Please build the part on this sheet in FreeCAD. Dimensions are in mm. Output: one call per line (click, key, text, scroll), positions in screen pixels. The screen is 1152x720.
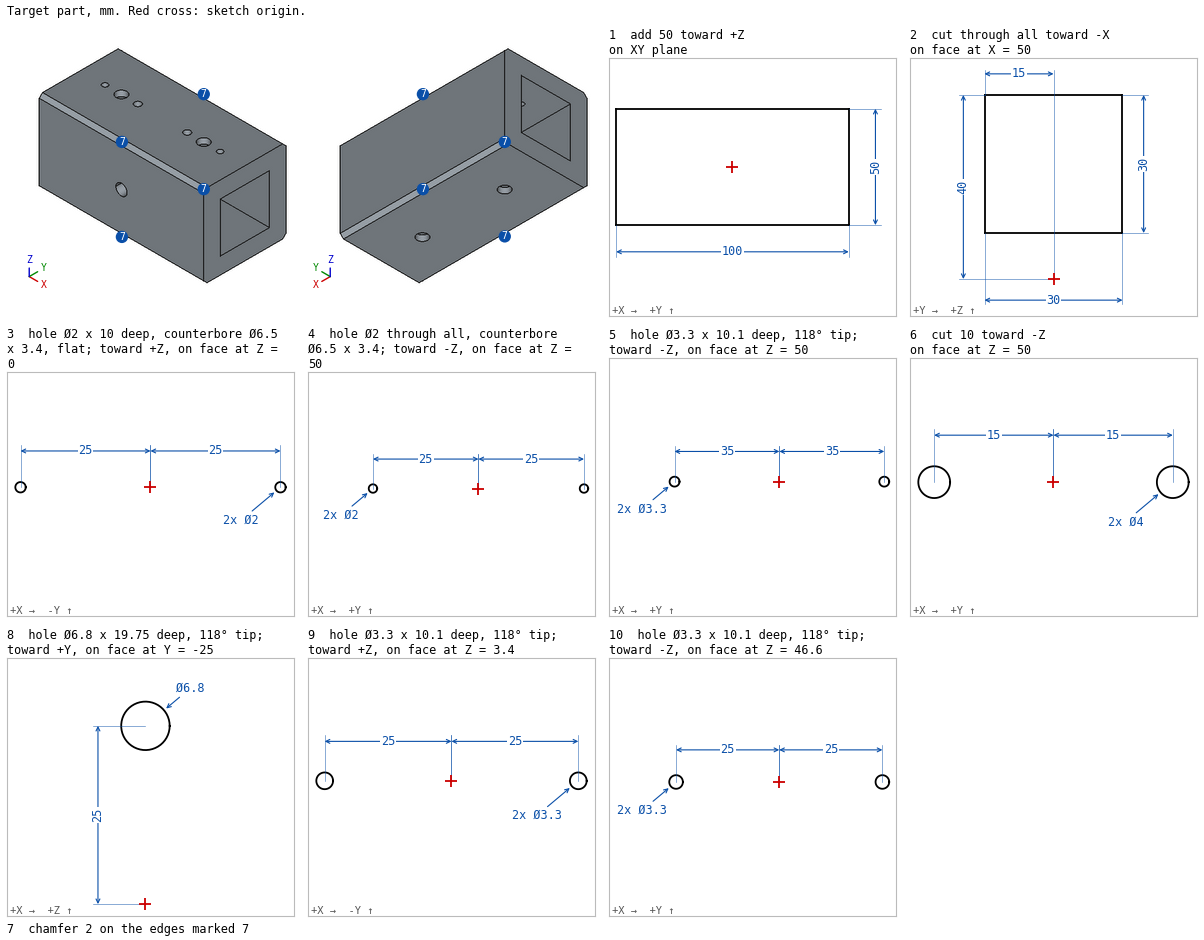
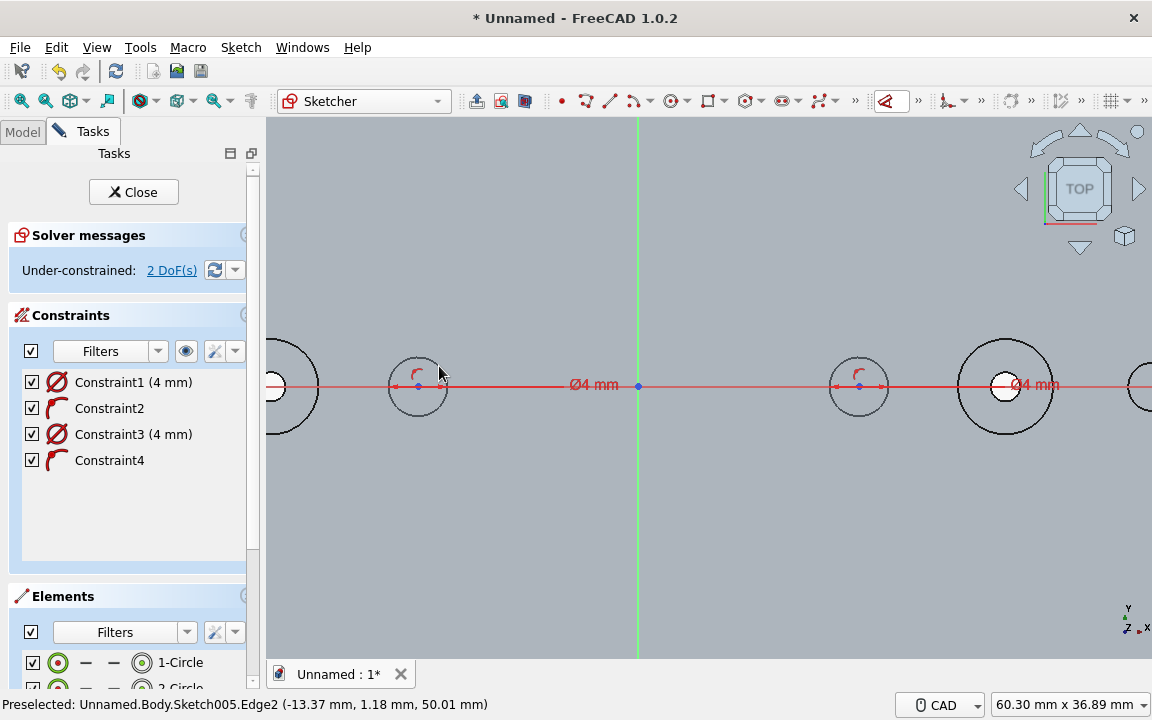
click(859, 387)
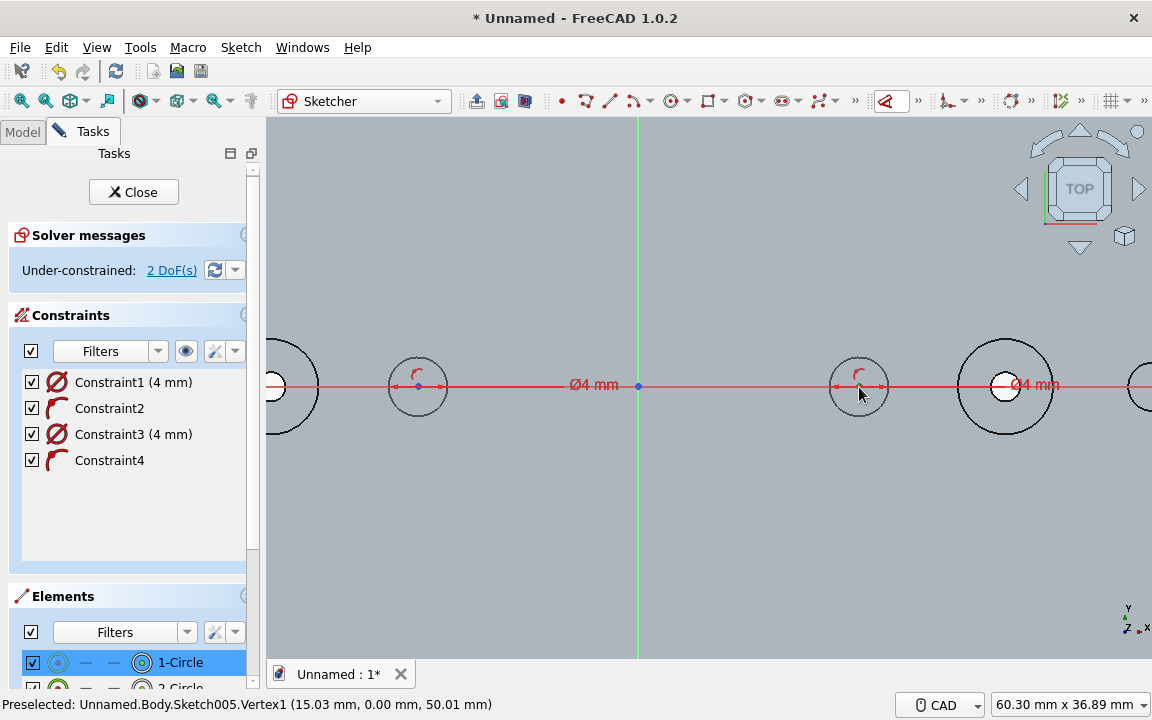
click(904, 102)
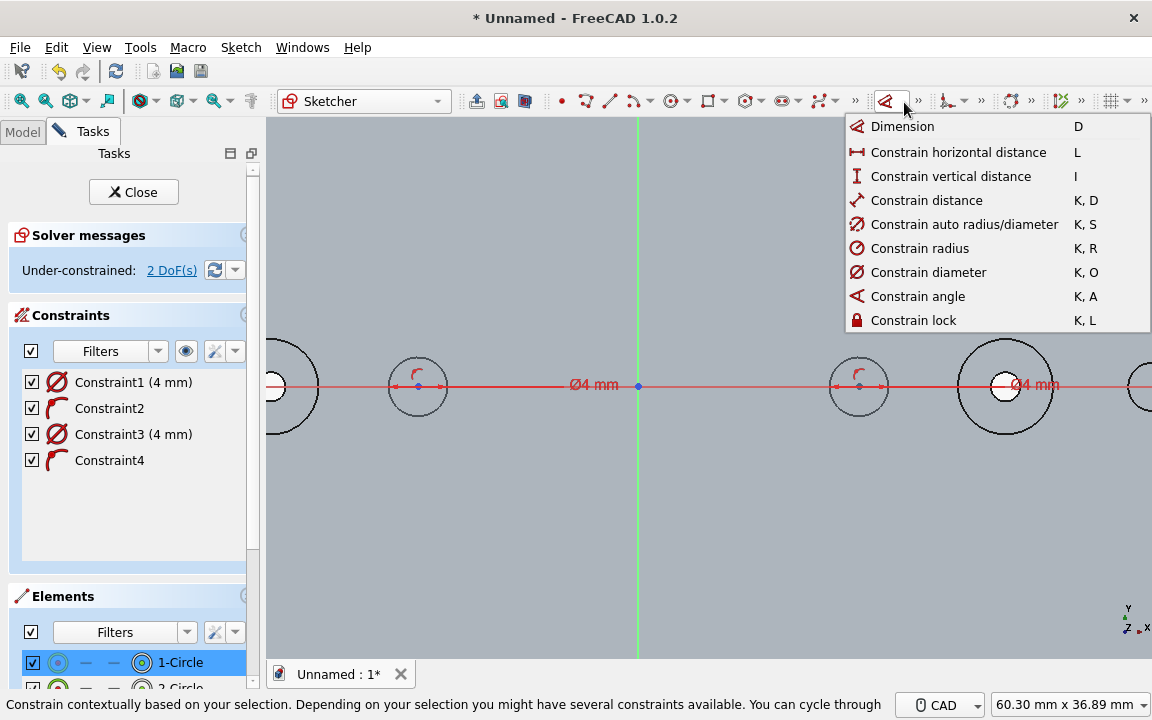
click(998, 152)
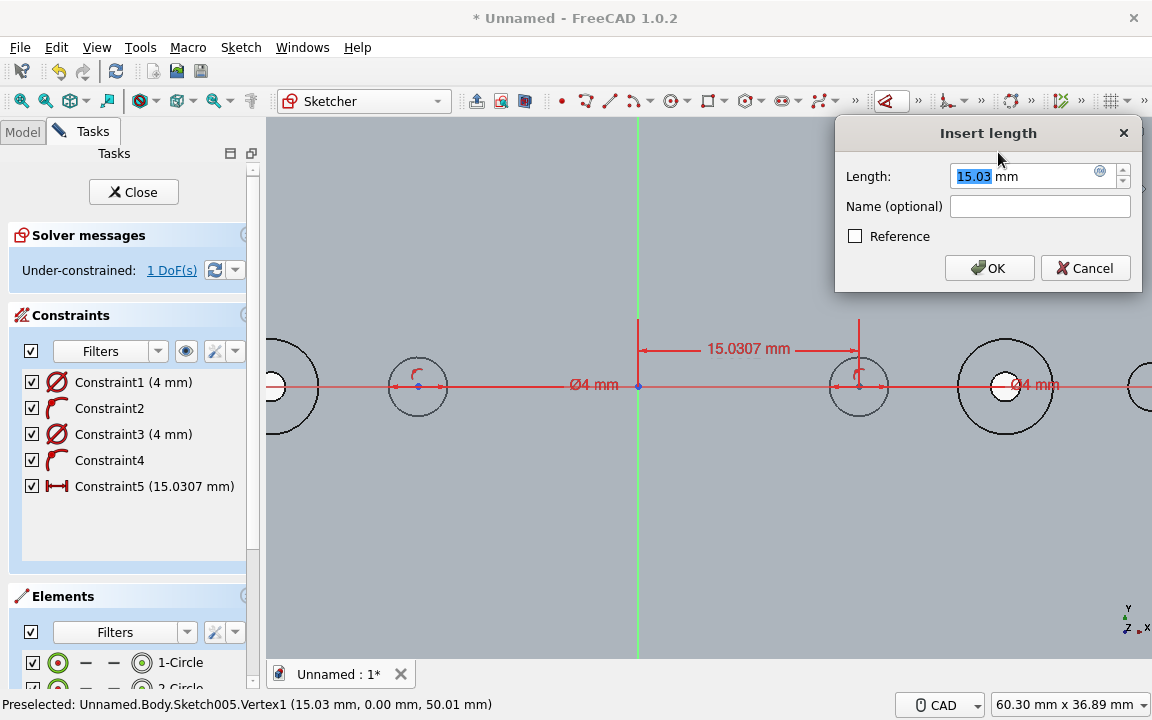
text(15)
key(Return)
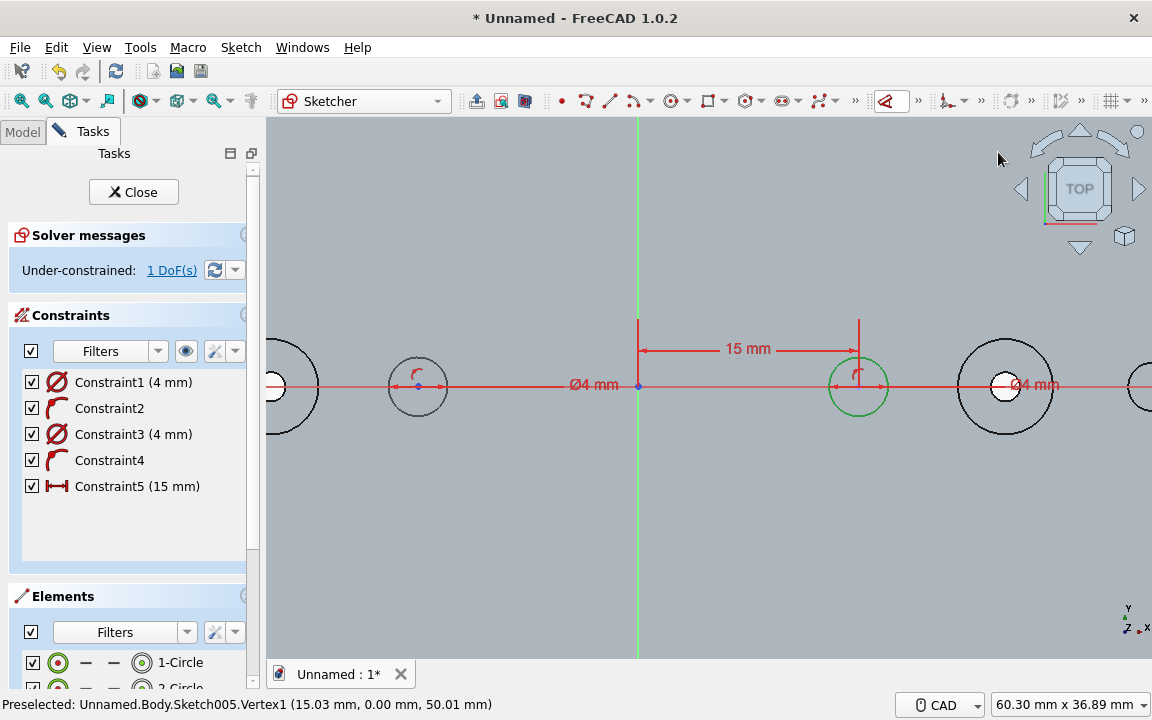
click(418, 387)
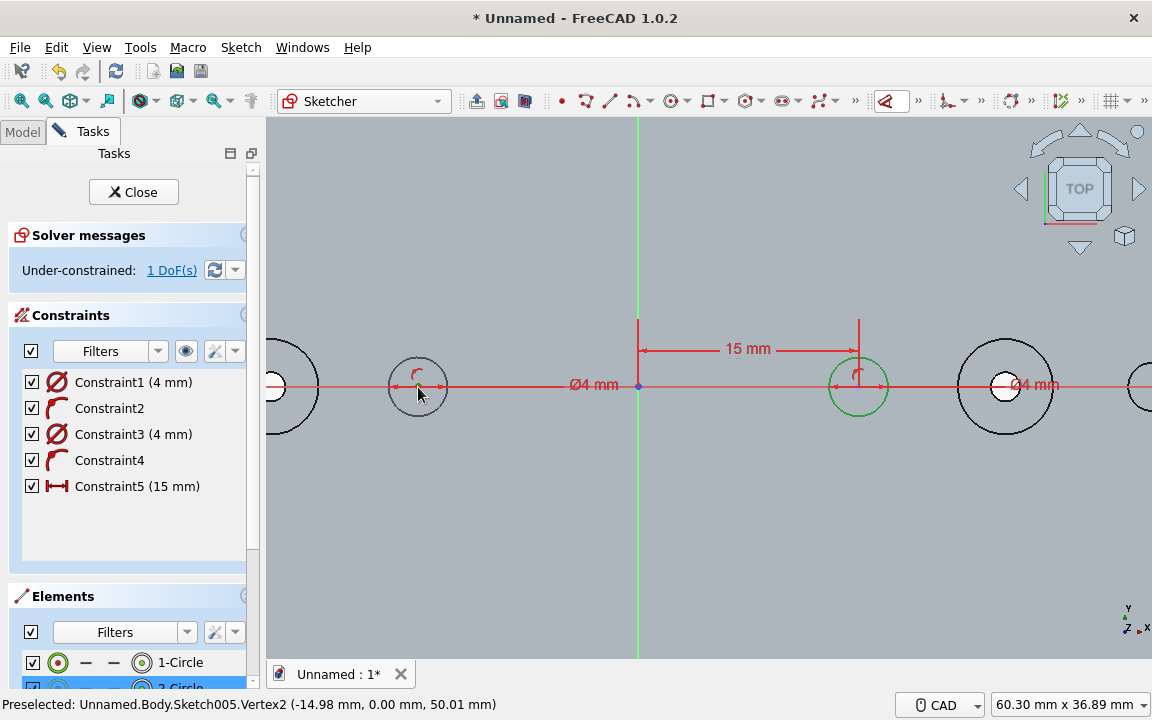
key(l)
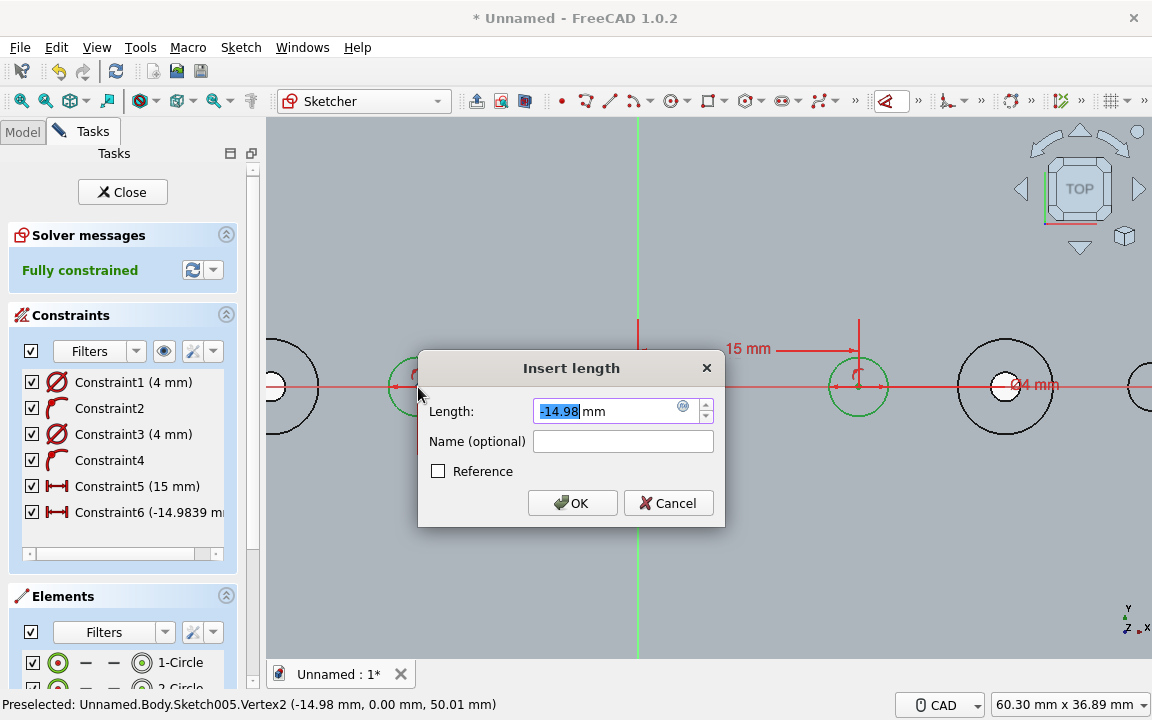
text(-15)
key(Return)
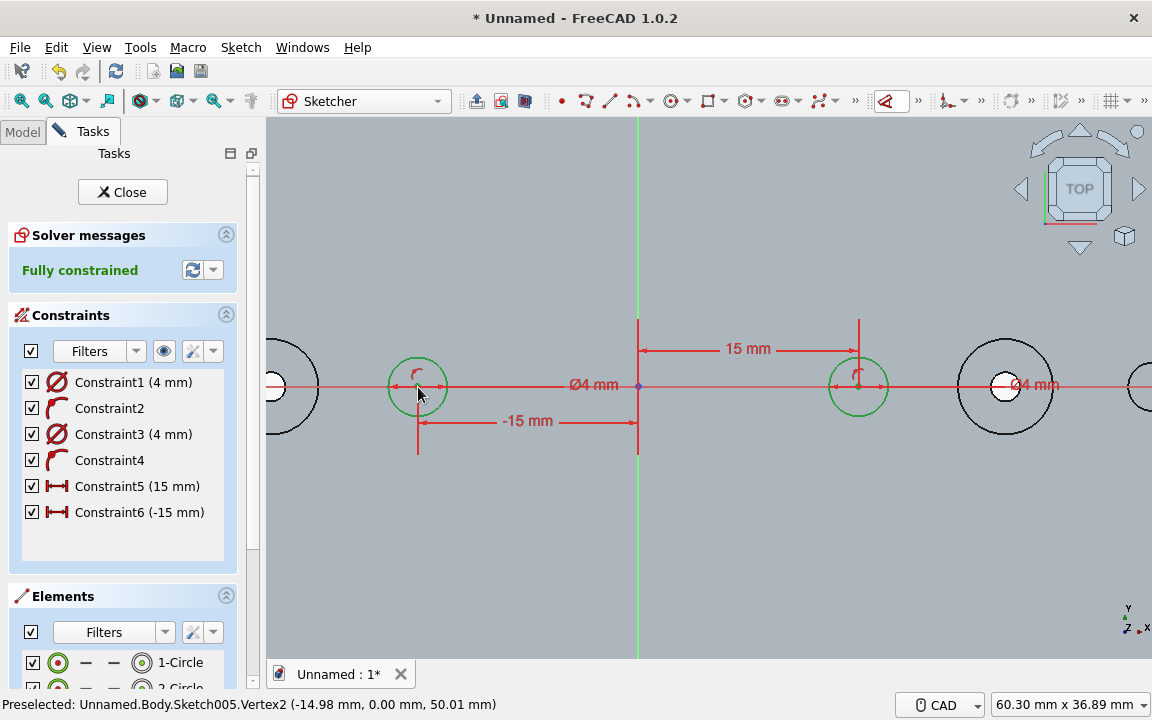
click(123, 192)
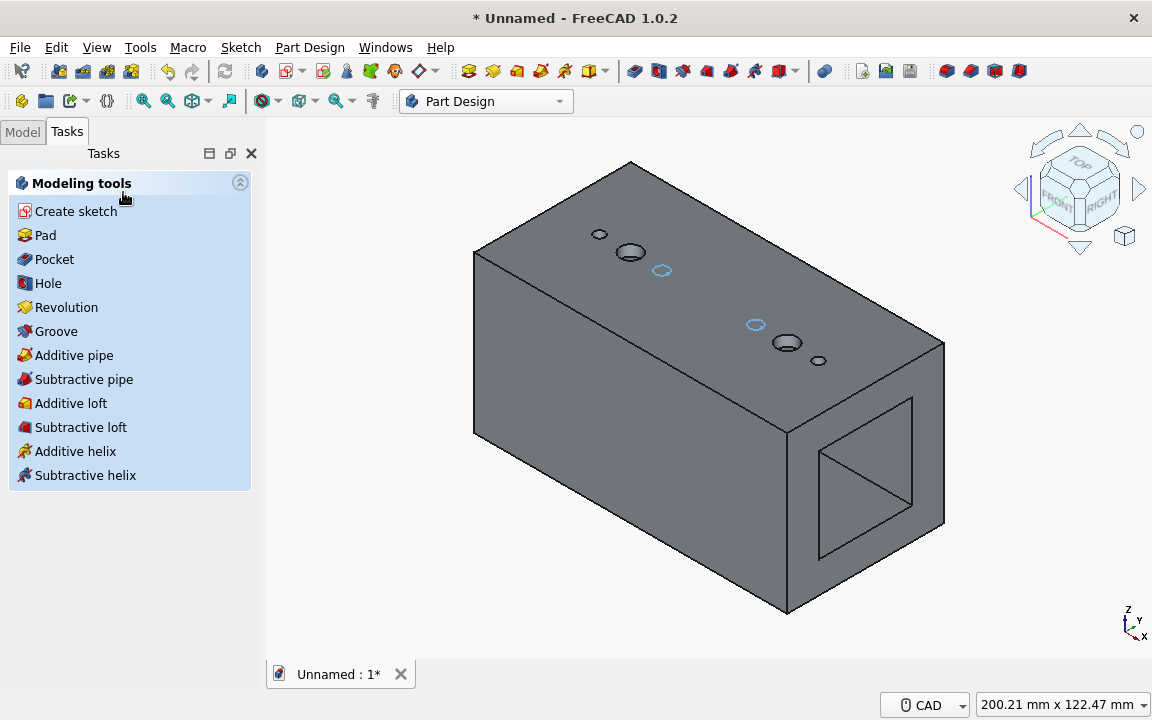
click(636, 72)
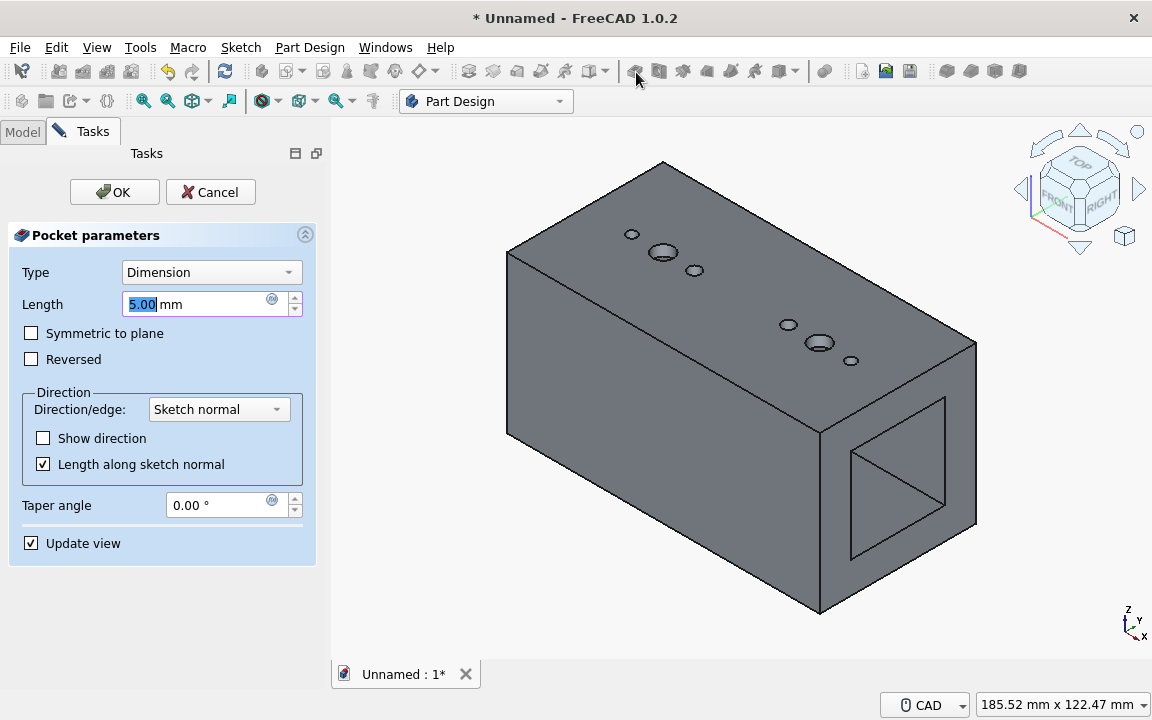
text(10)
key(Tab)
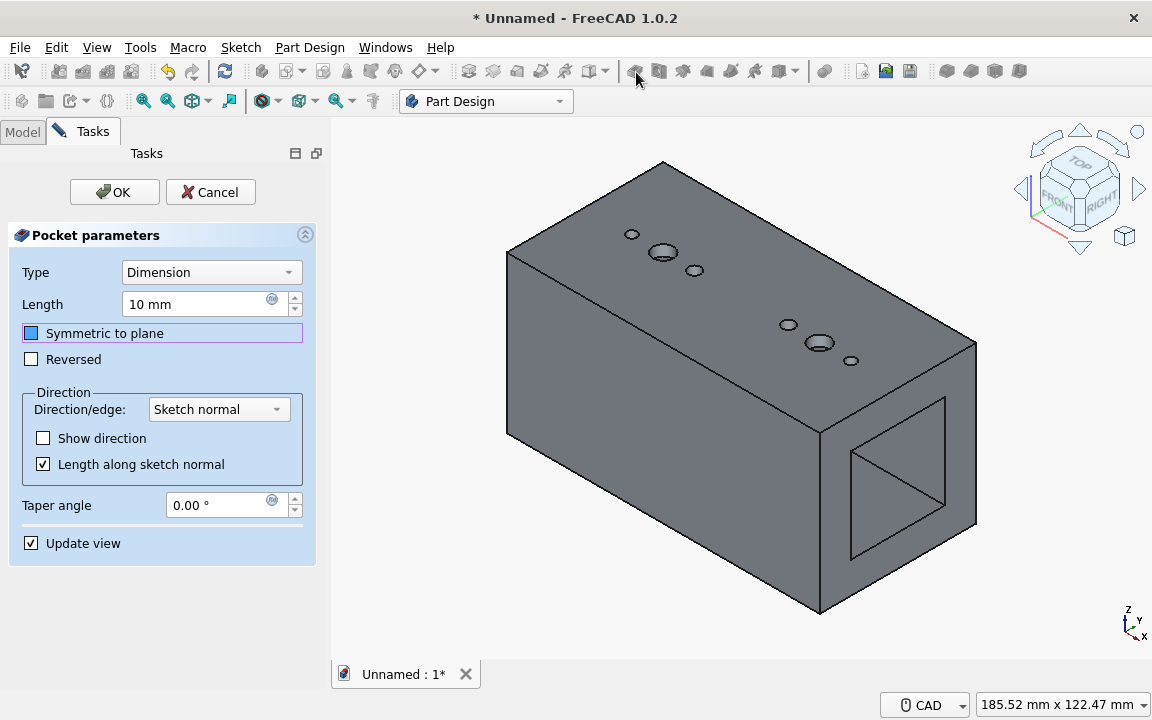
click(115, 192)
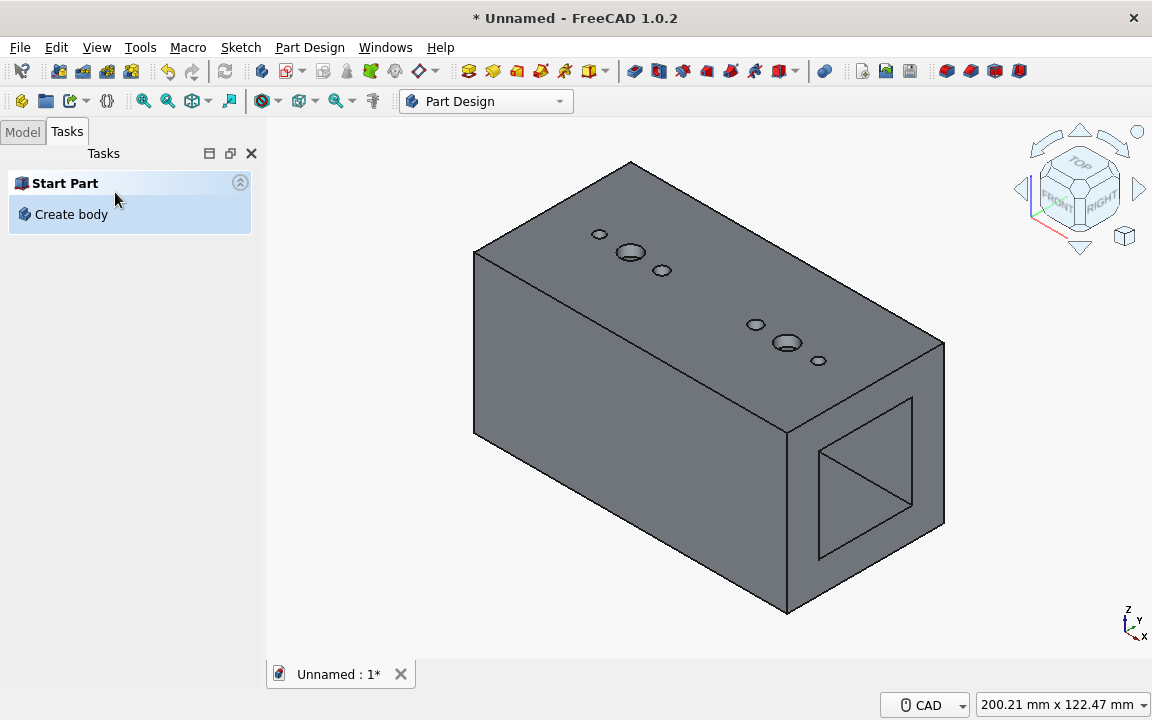
click(631, 342)